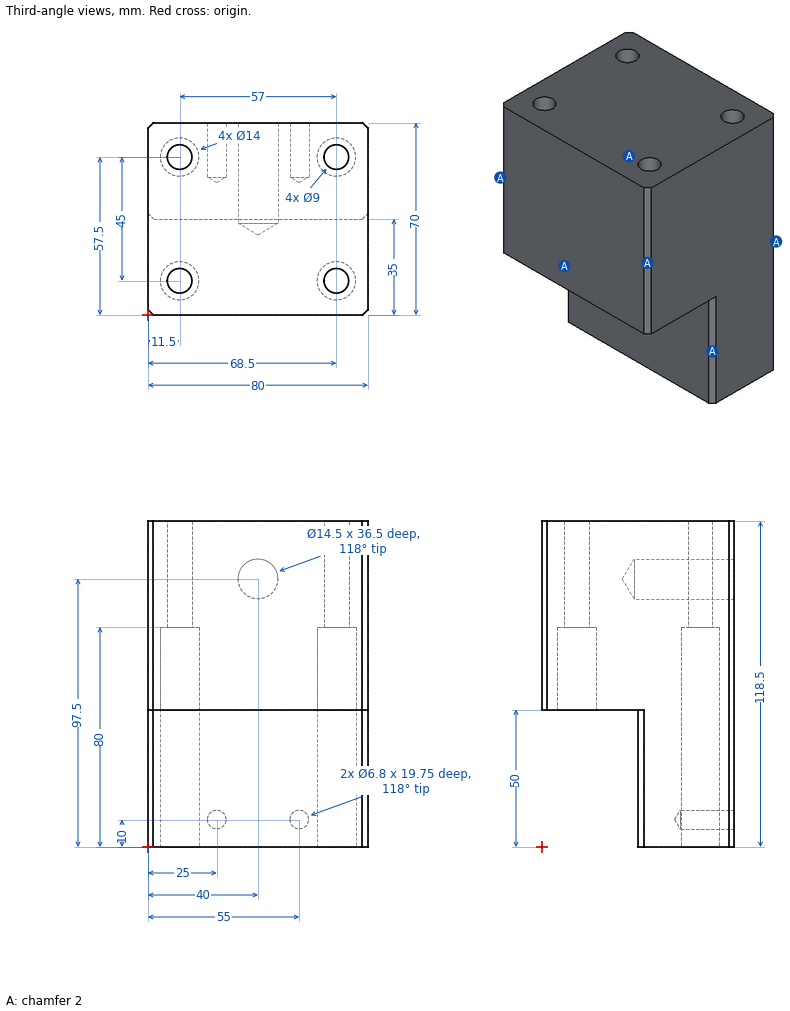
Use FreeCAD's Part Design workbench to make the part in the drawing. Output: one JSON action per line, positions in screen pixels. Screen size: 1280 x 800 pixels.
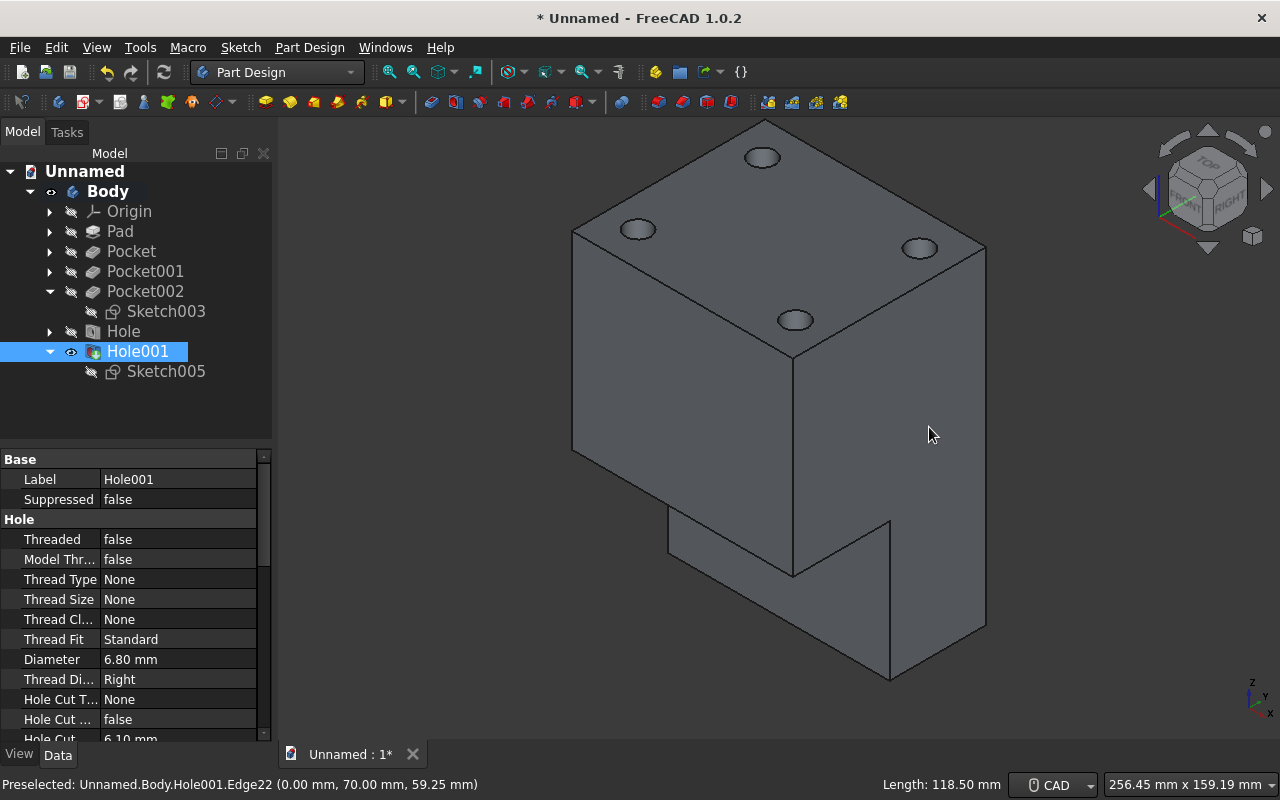
{"action": "left_click", "coordinate": [890, 600], "text": "ctrl"}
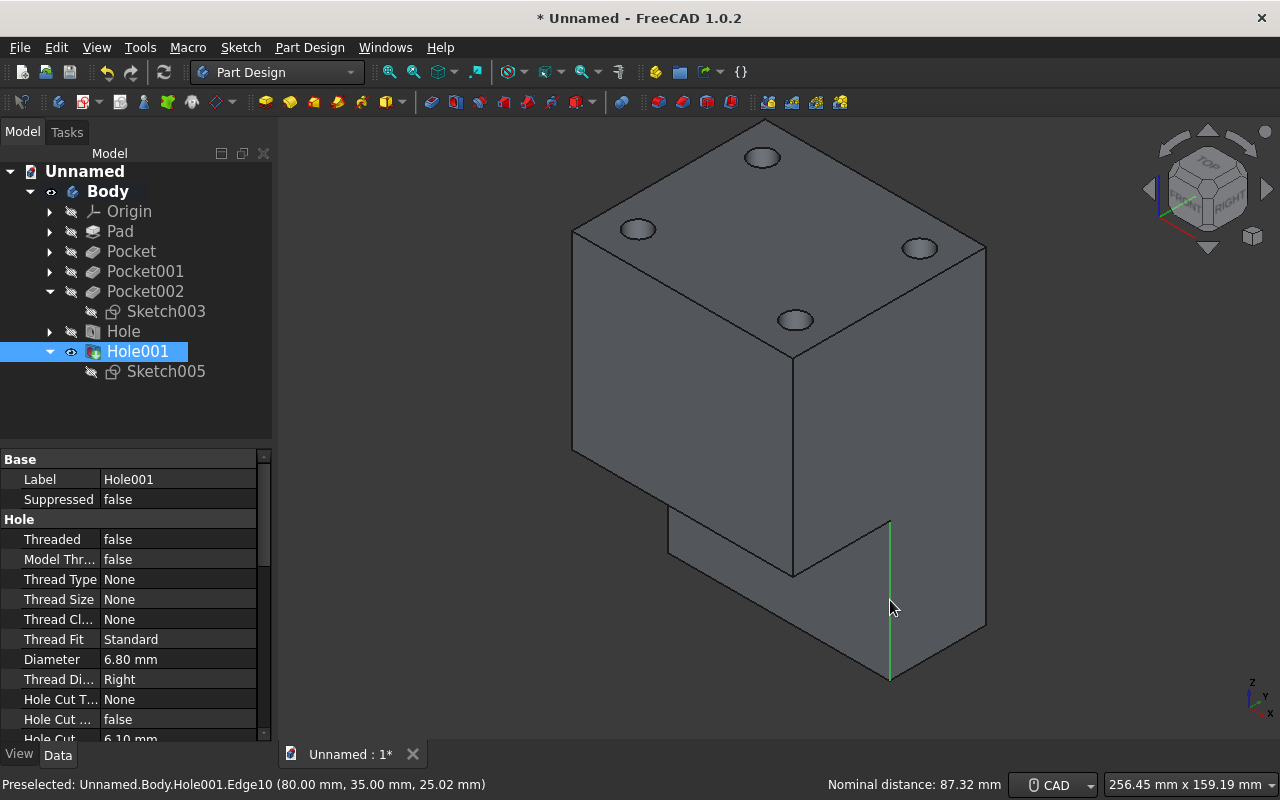
{"action": "left_click", "coordinate": [793, 467], "text": "ctrl"}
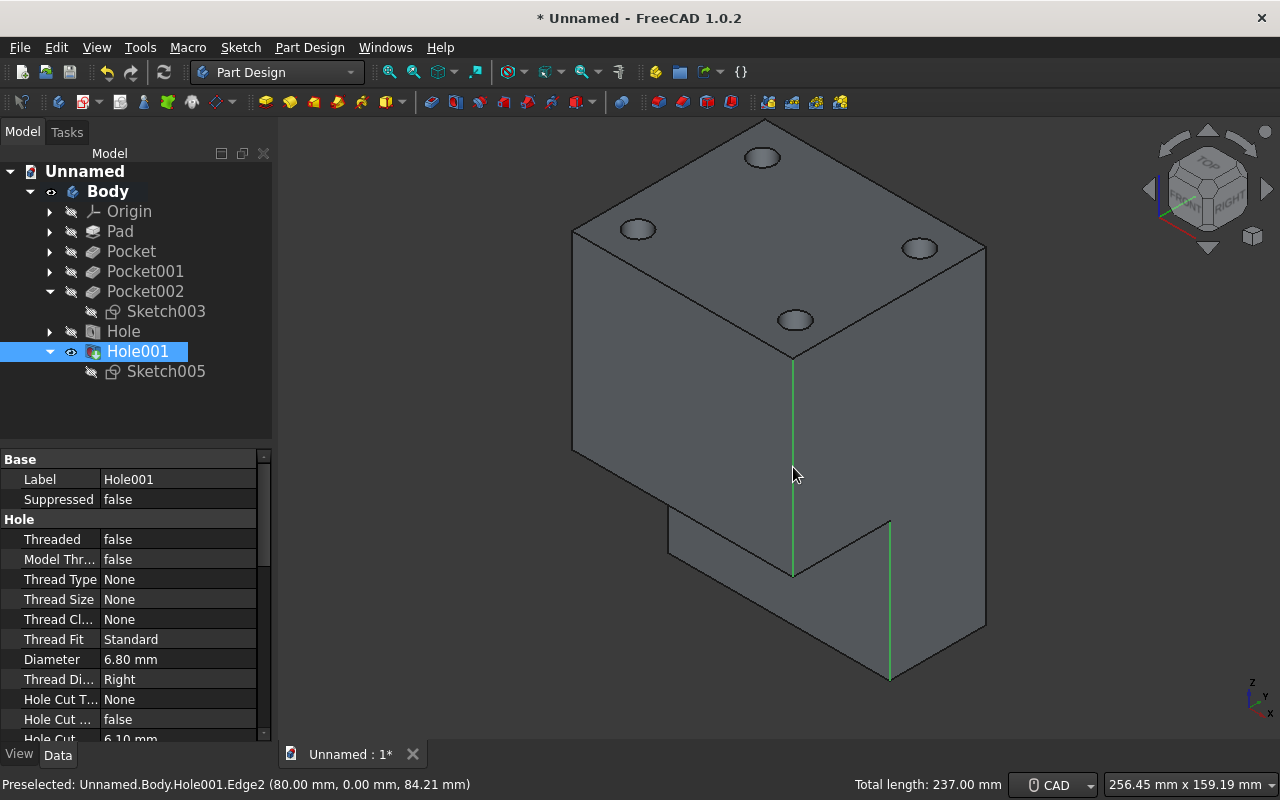
{"action": "key", "text": "2"}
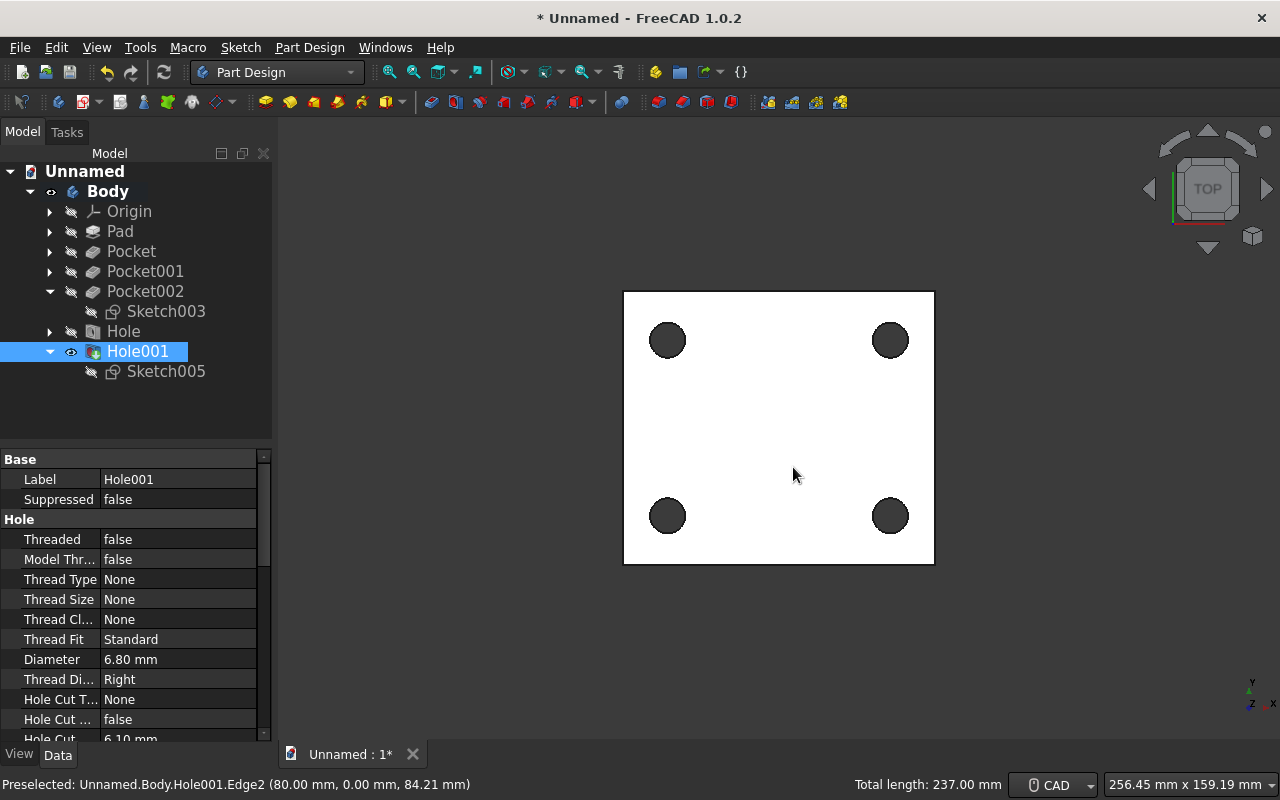
{"action": "key", "text": "v f"}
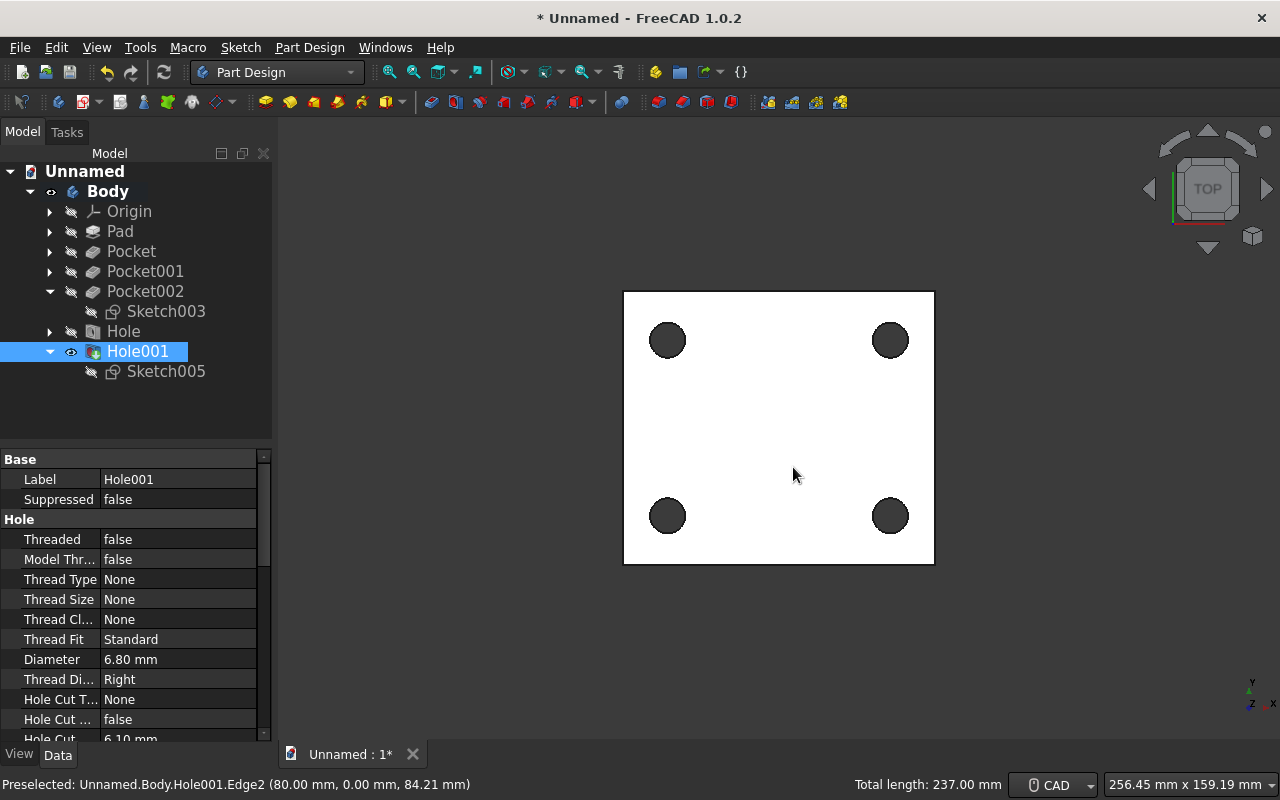
{"action": "key", "text": "1"}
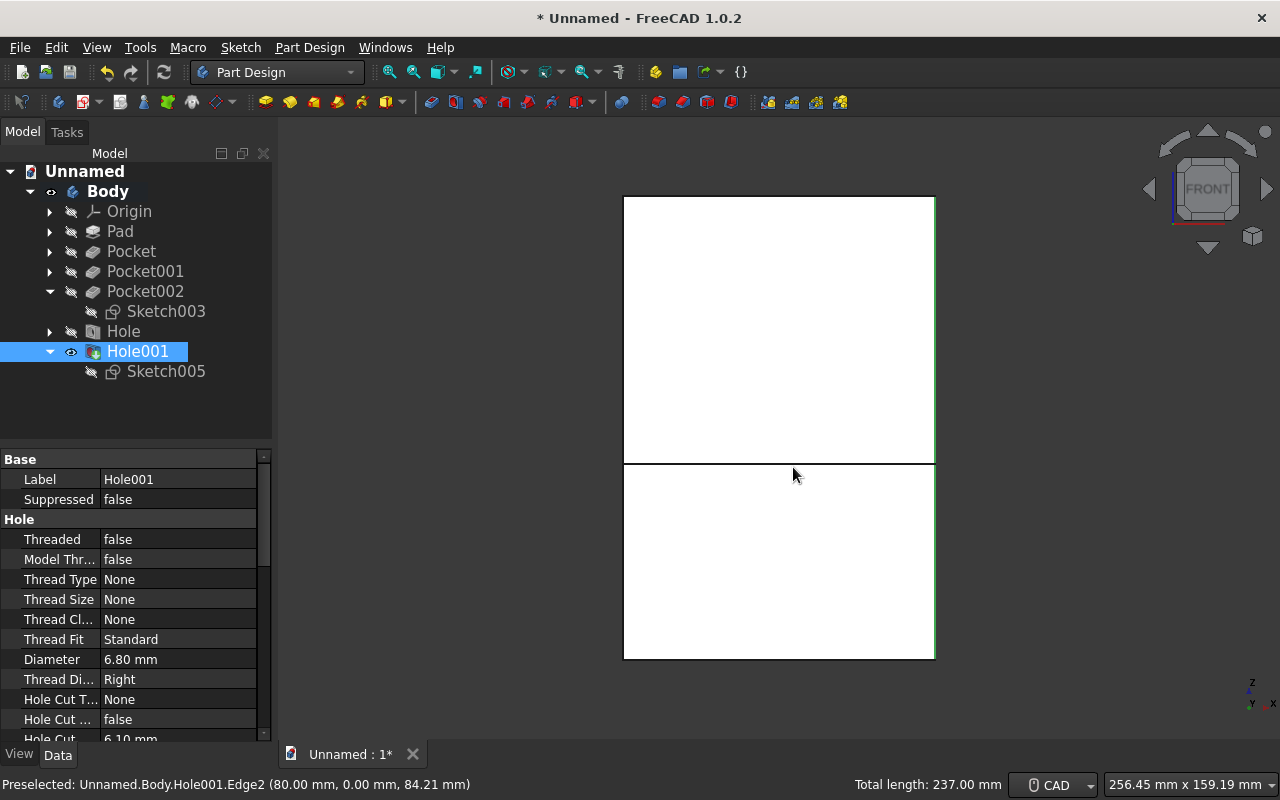
{"action": "left_click", "coordinate": [623, 561], "text": "ctrl"}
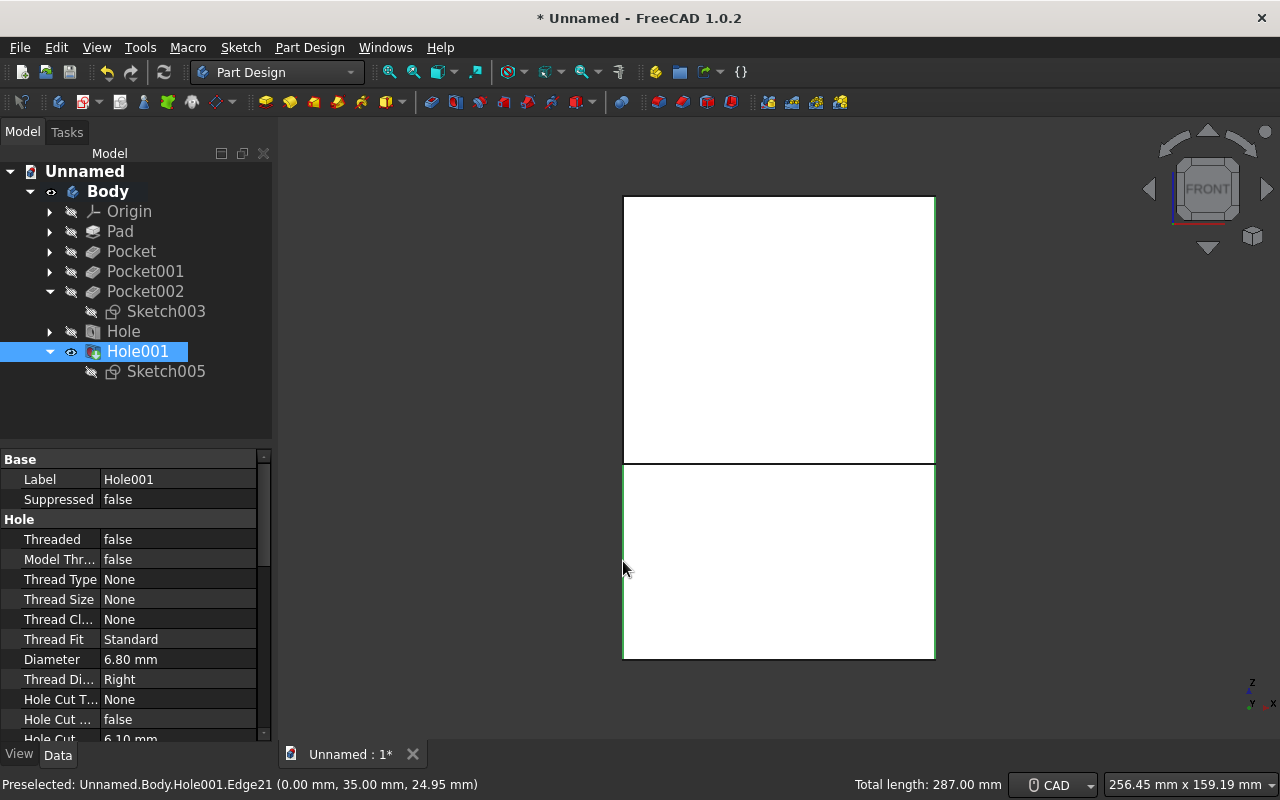
{"action": "left_click", "coordinate": [623, 329], "text": "ctrl"}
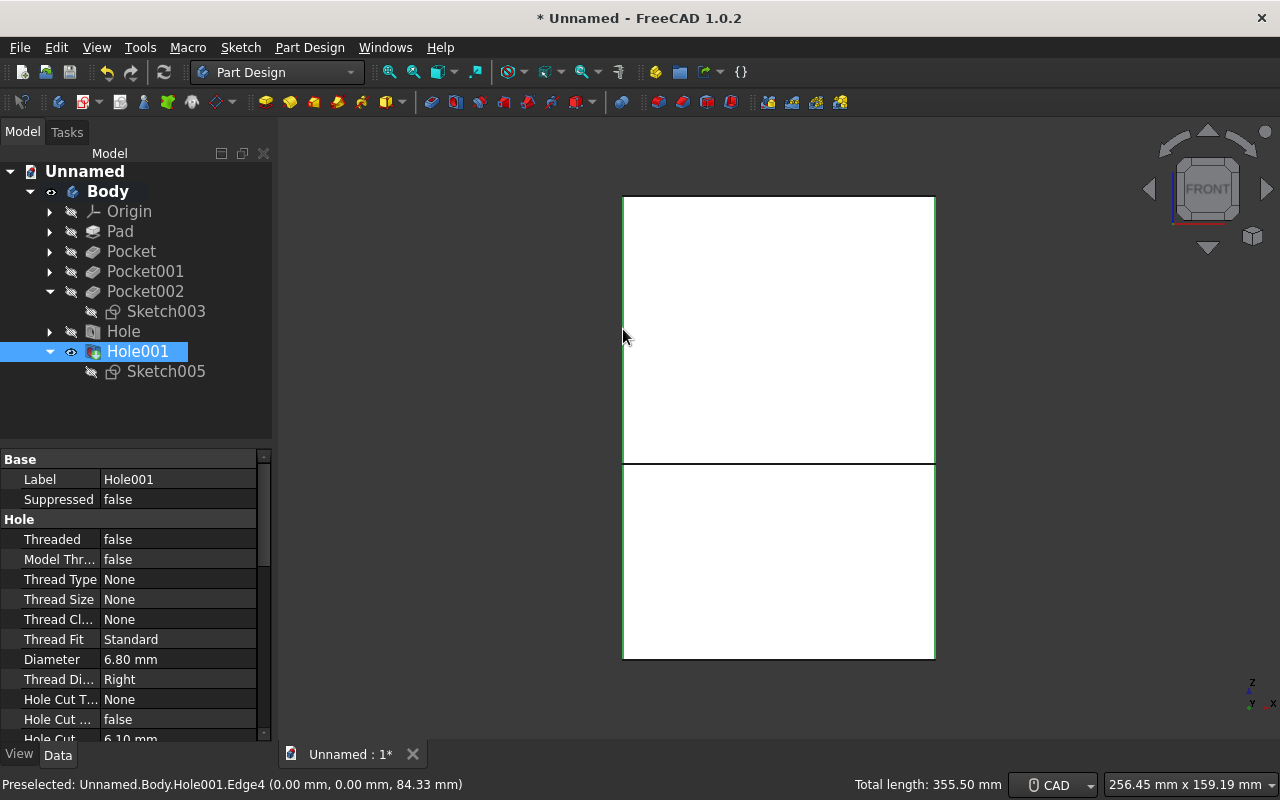
{"action": "key", "text": "3"}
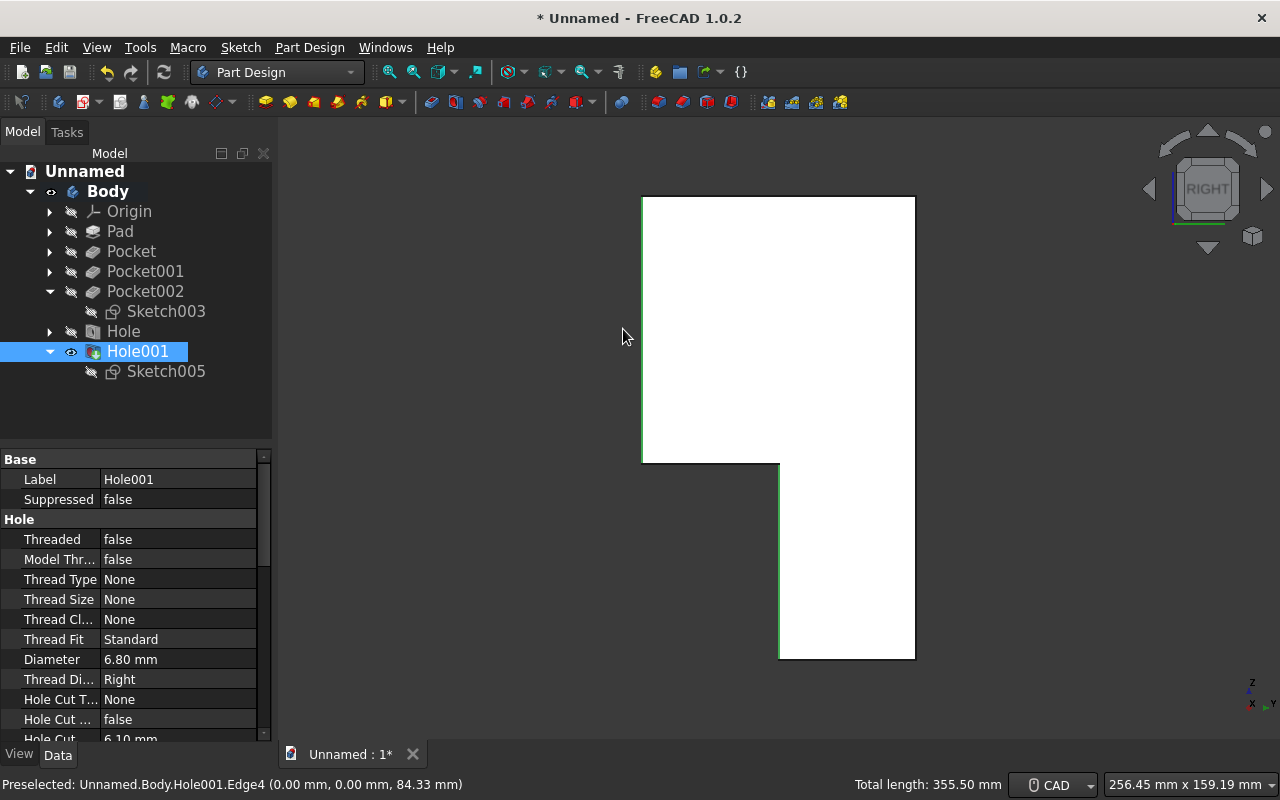
{"action": "left_click", "coordinate": [916, 427], "text": "ctrl"}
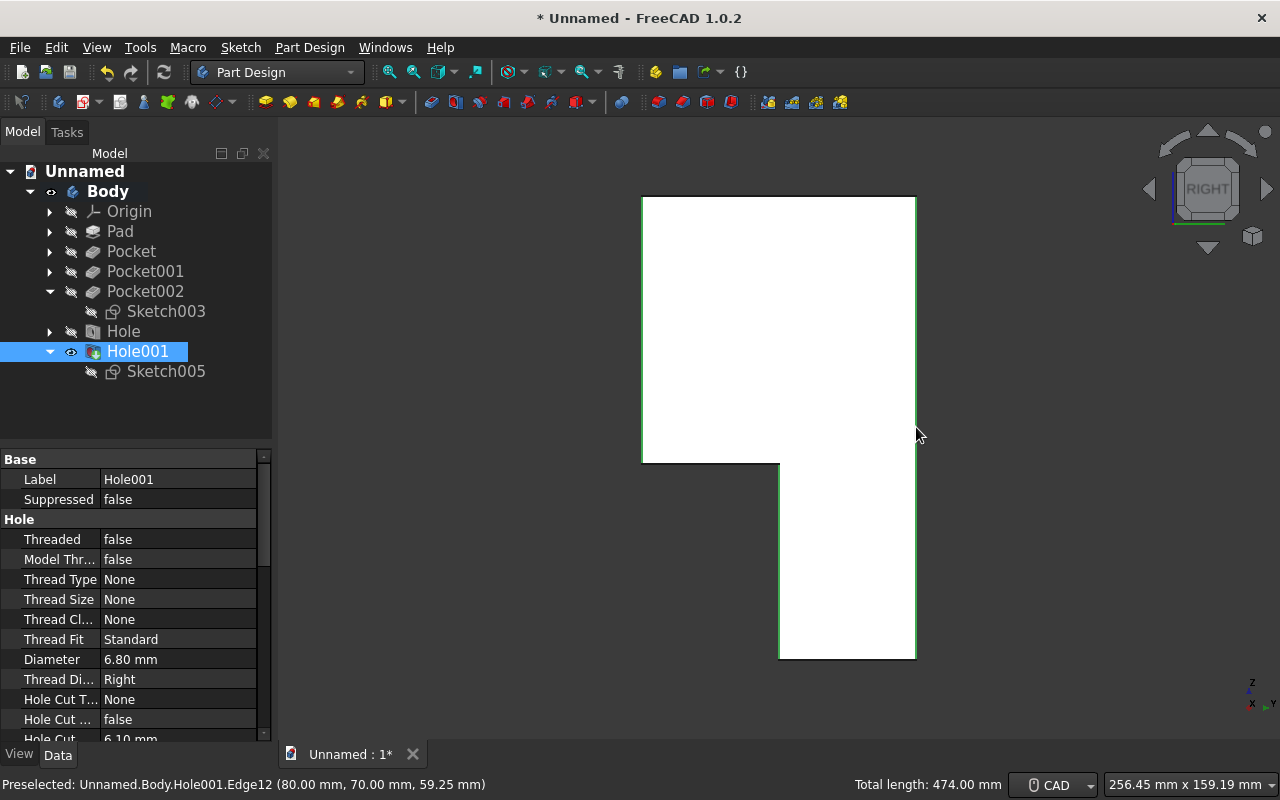
{"action": "left_click", "coordinate": [684, 102]}